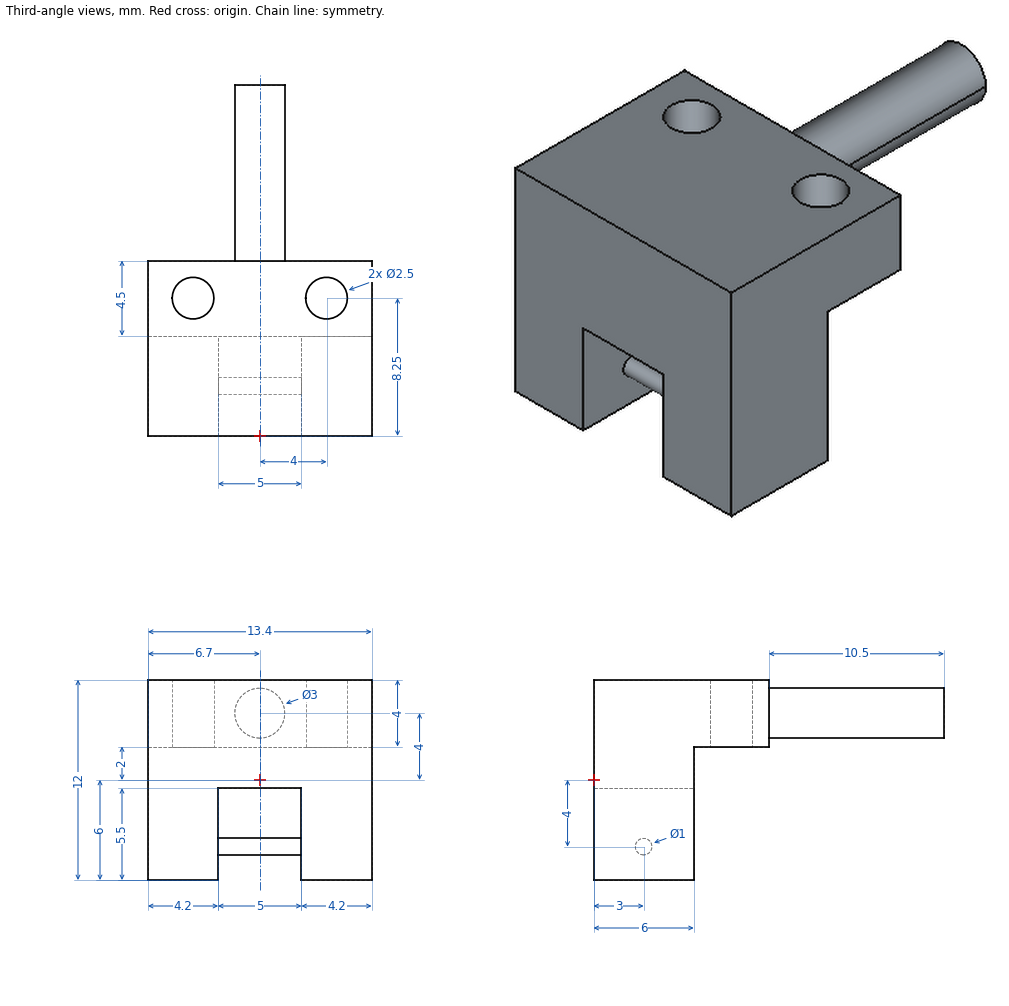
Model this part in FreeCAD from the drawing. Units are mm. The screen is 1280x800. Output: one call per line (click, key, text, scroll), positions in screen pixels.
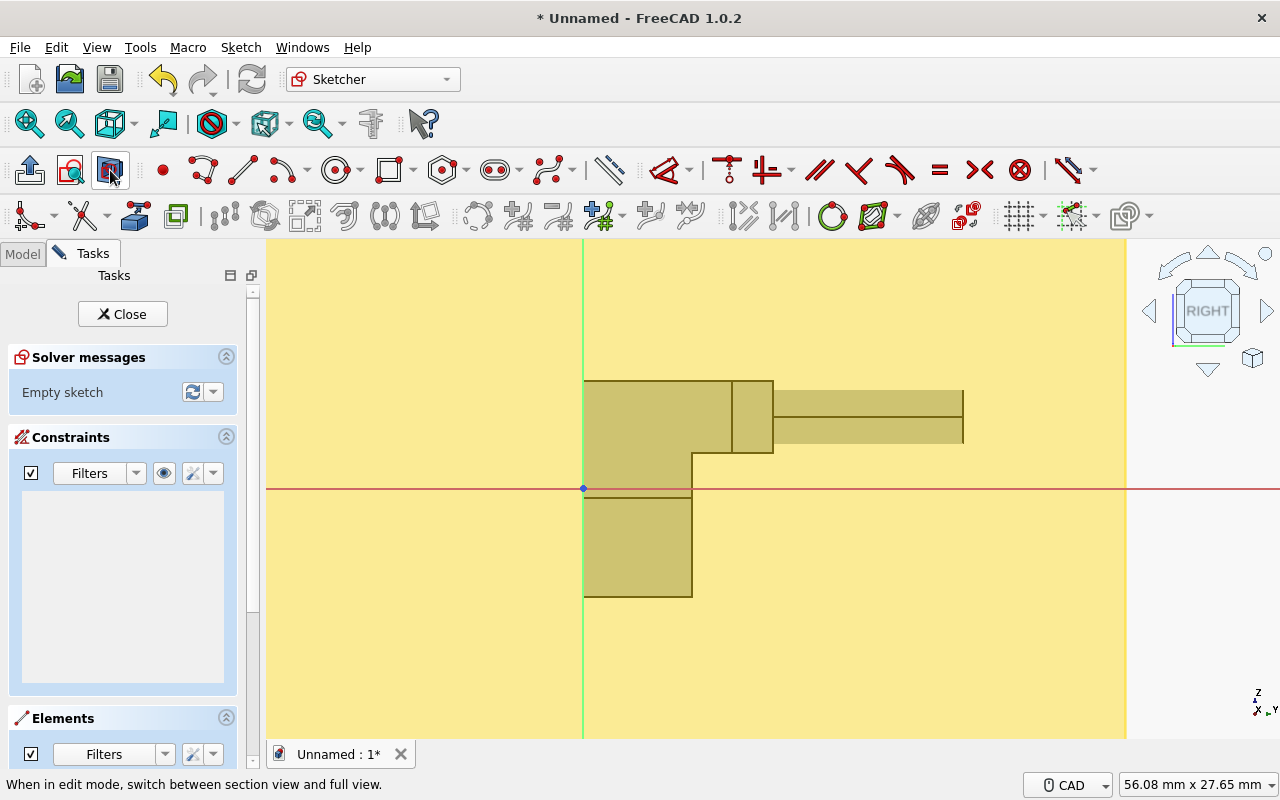
scroll(633, 566, up, 14)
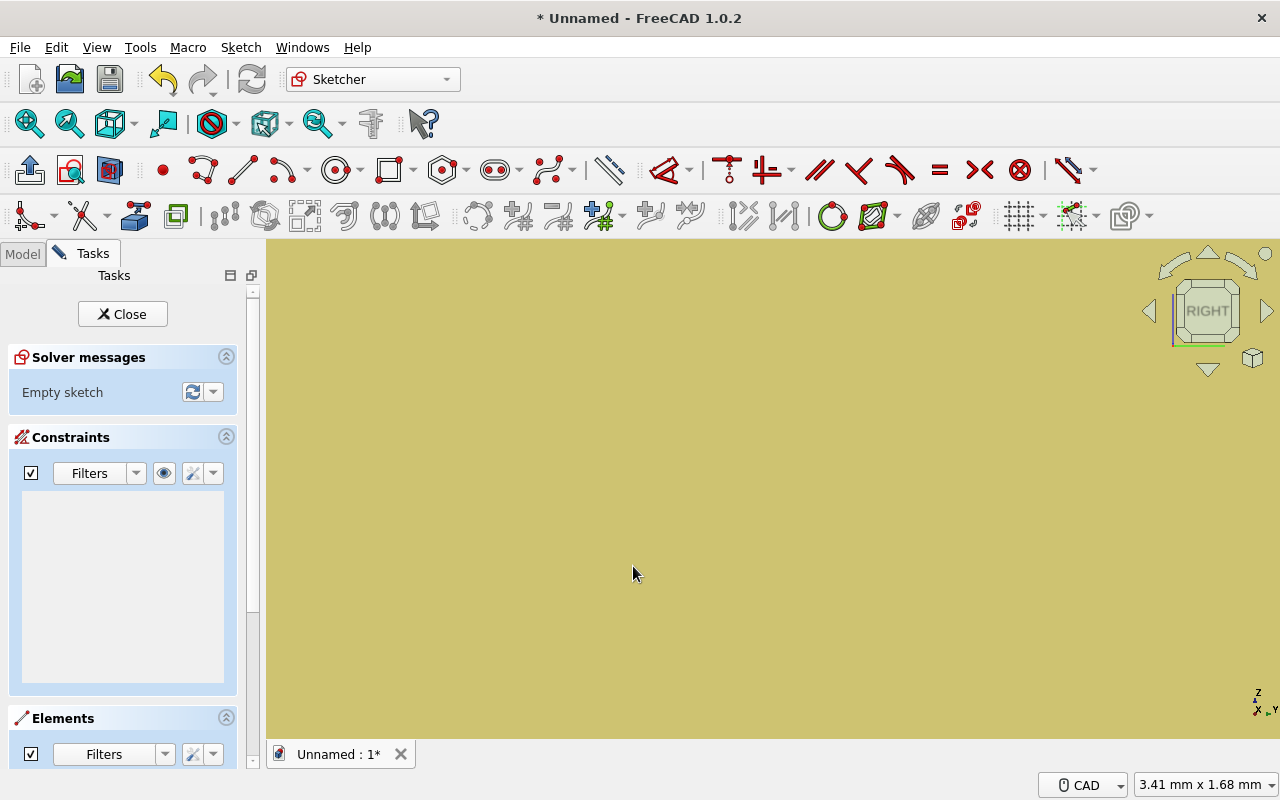
click(336, 170)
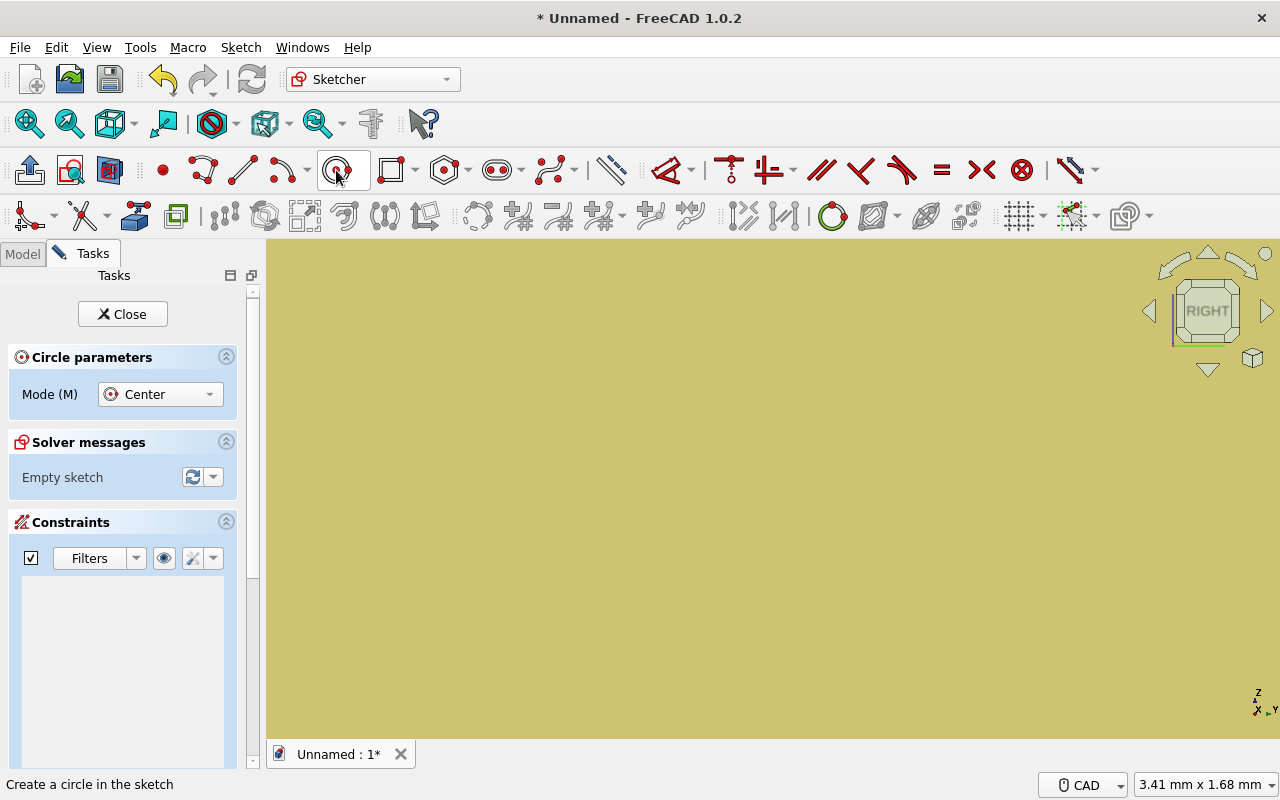
click(699, 479)
move(805, 374)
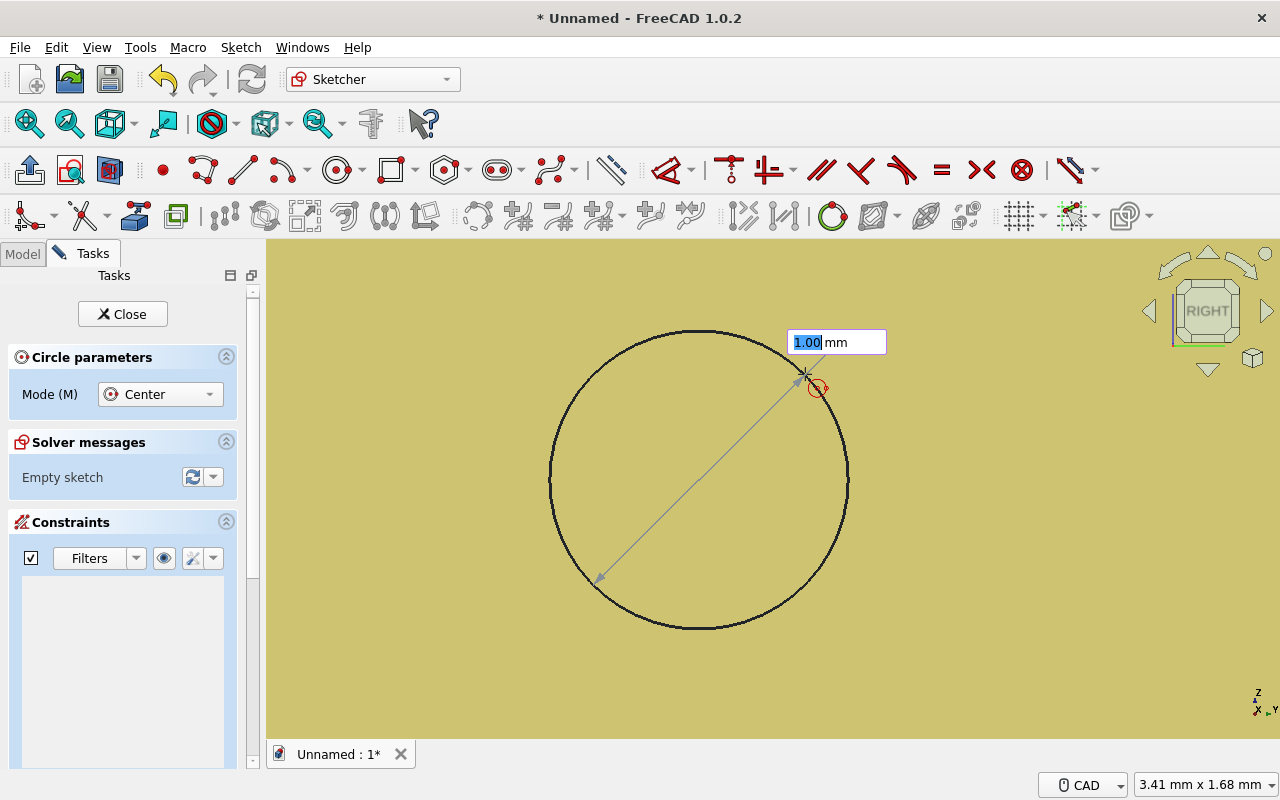
text(1)
key(Return)
key(Escape)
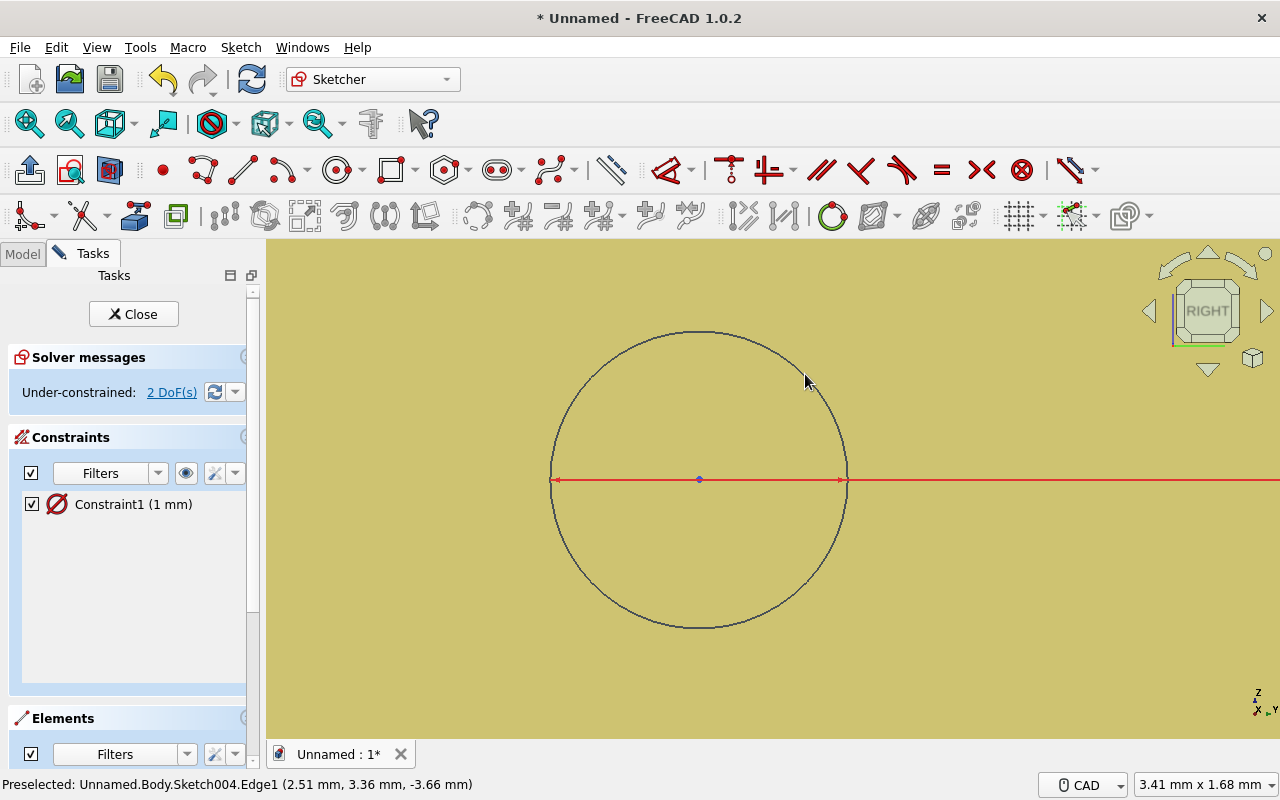
click(666, 170)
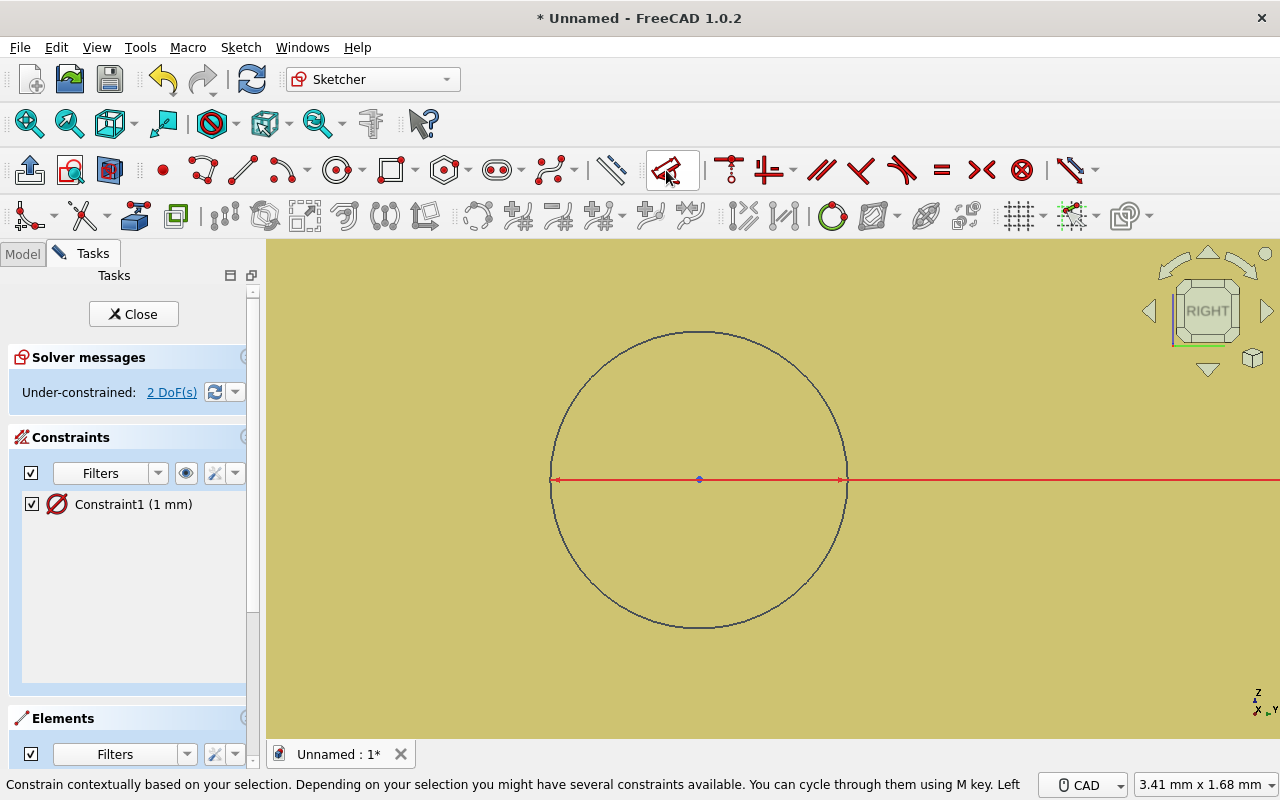
click(699, 480)
click(497, 514)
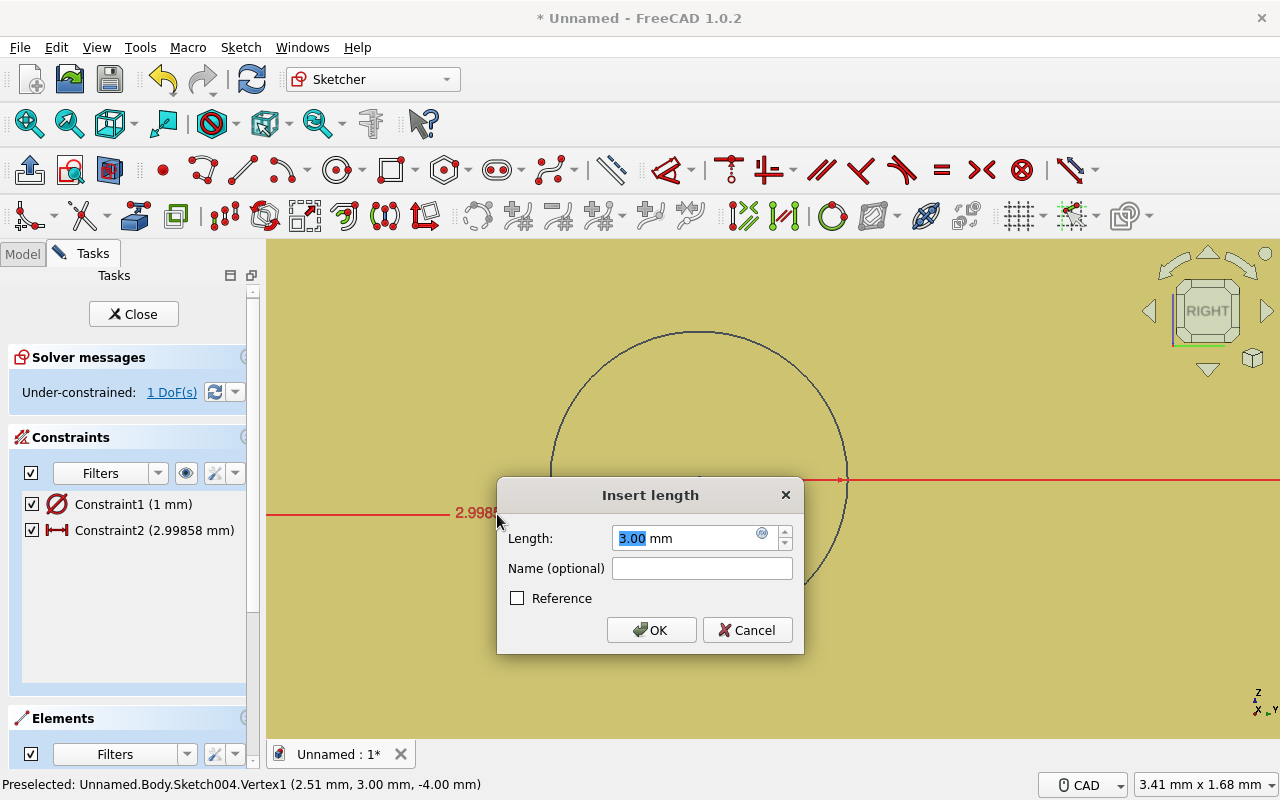
text(3)
key(Return)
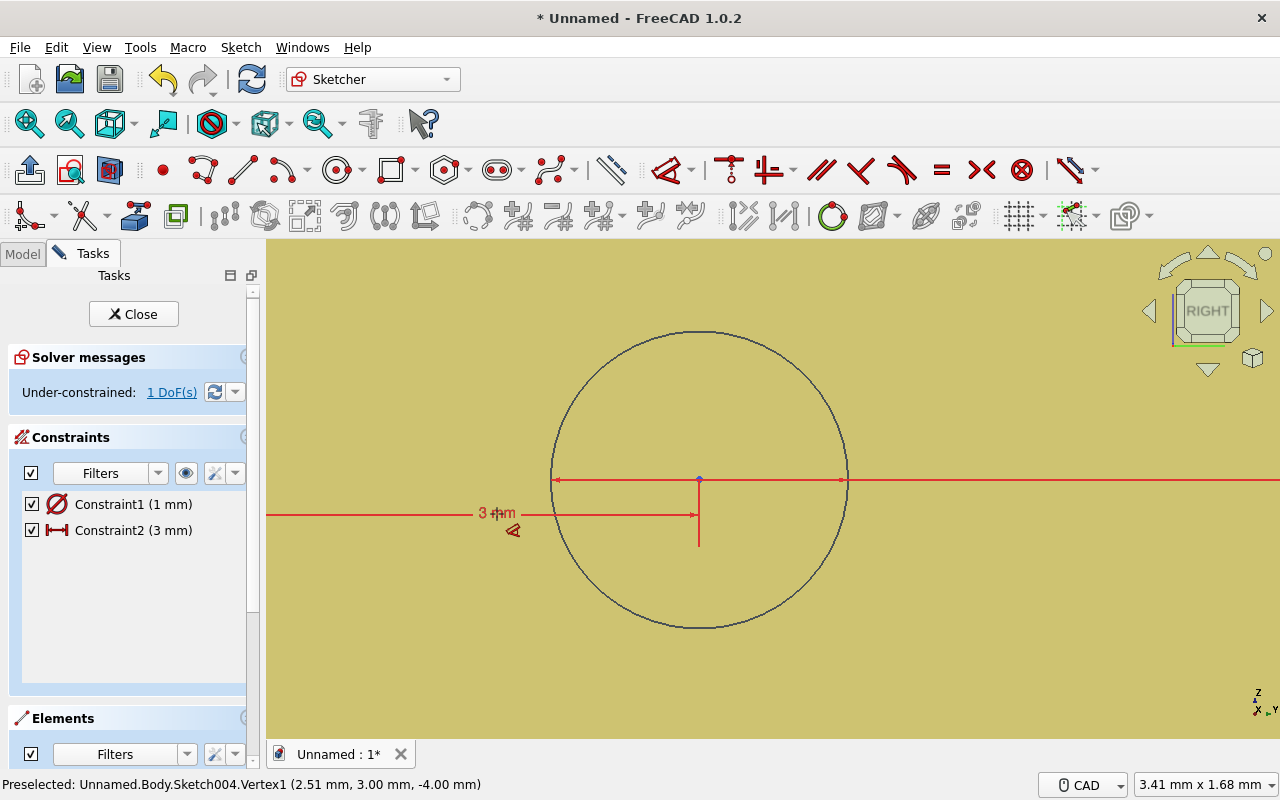
click(699, 480)
click(733, 373)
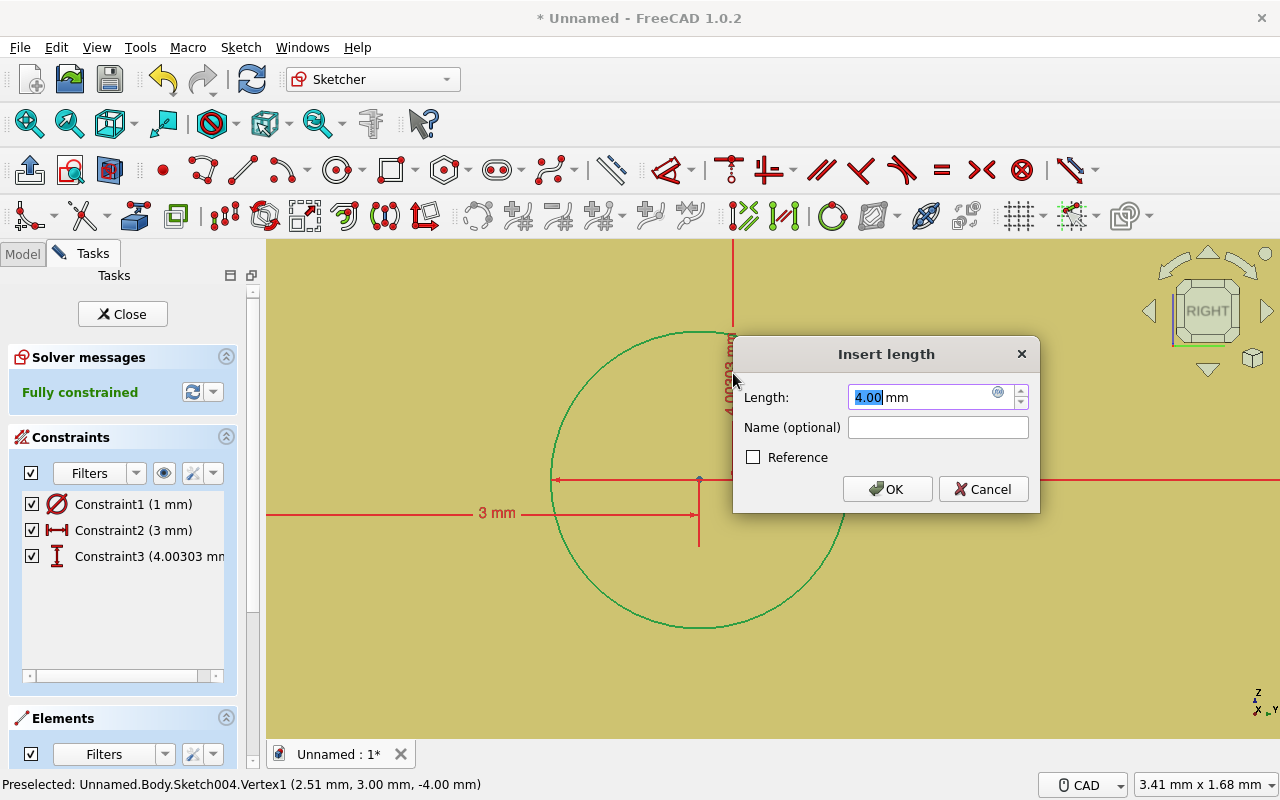
text(4)
key(Return)
key(Escape)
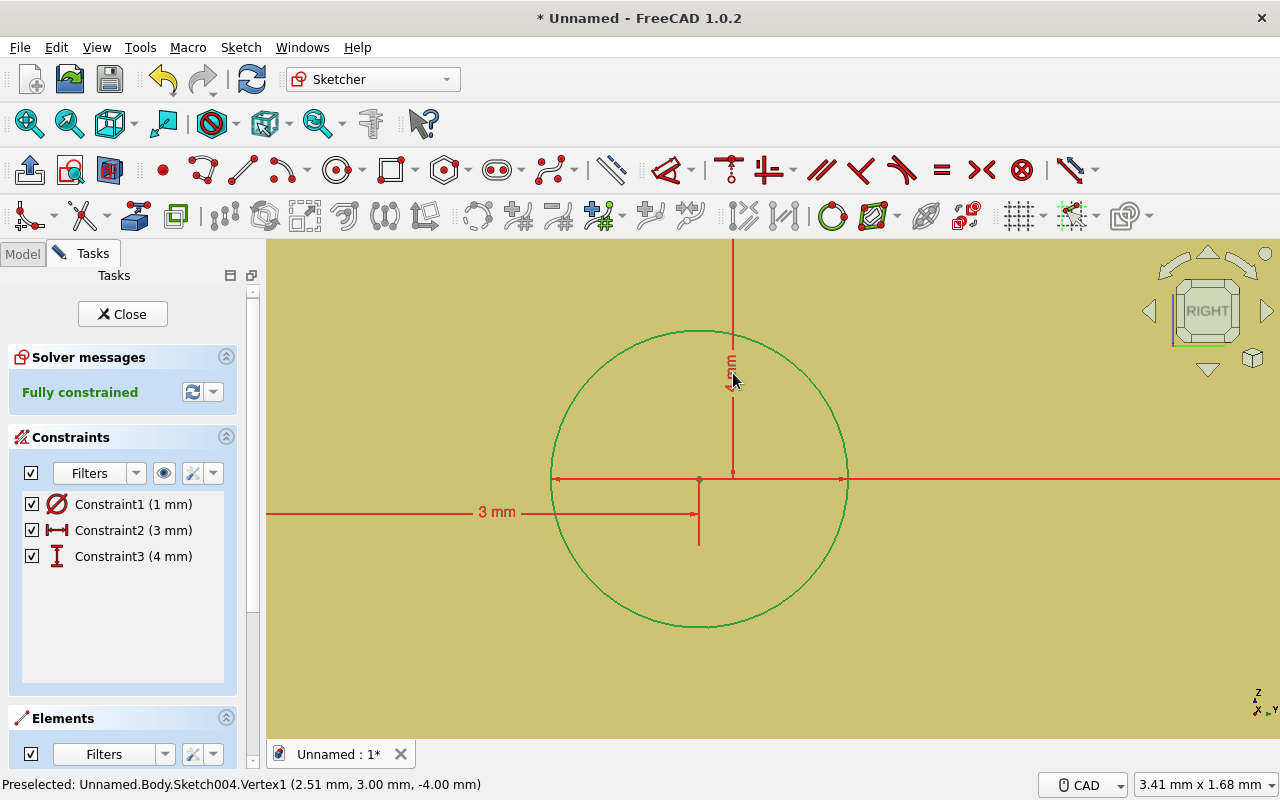
click(123, 314)